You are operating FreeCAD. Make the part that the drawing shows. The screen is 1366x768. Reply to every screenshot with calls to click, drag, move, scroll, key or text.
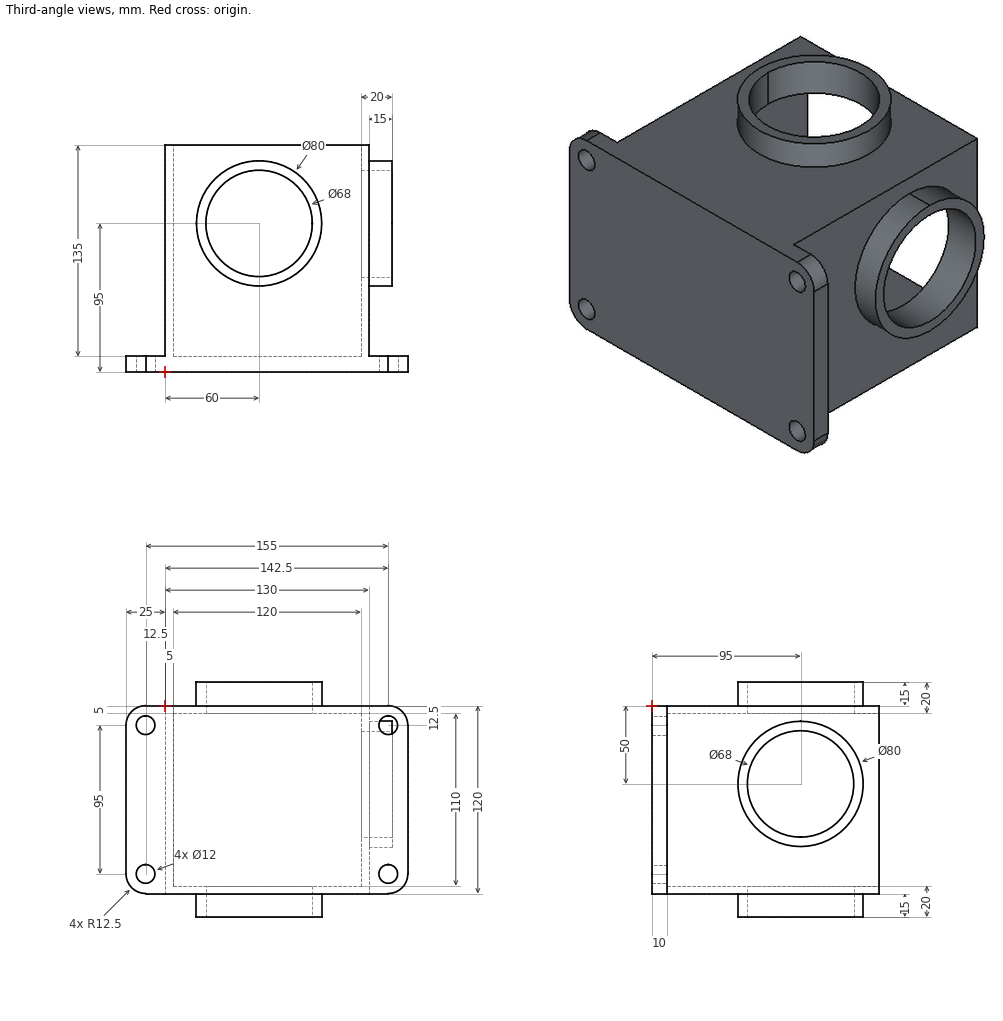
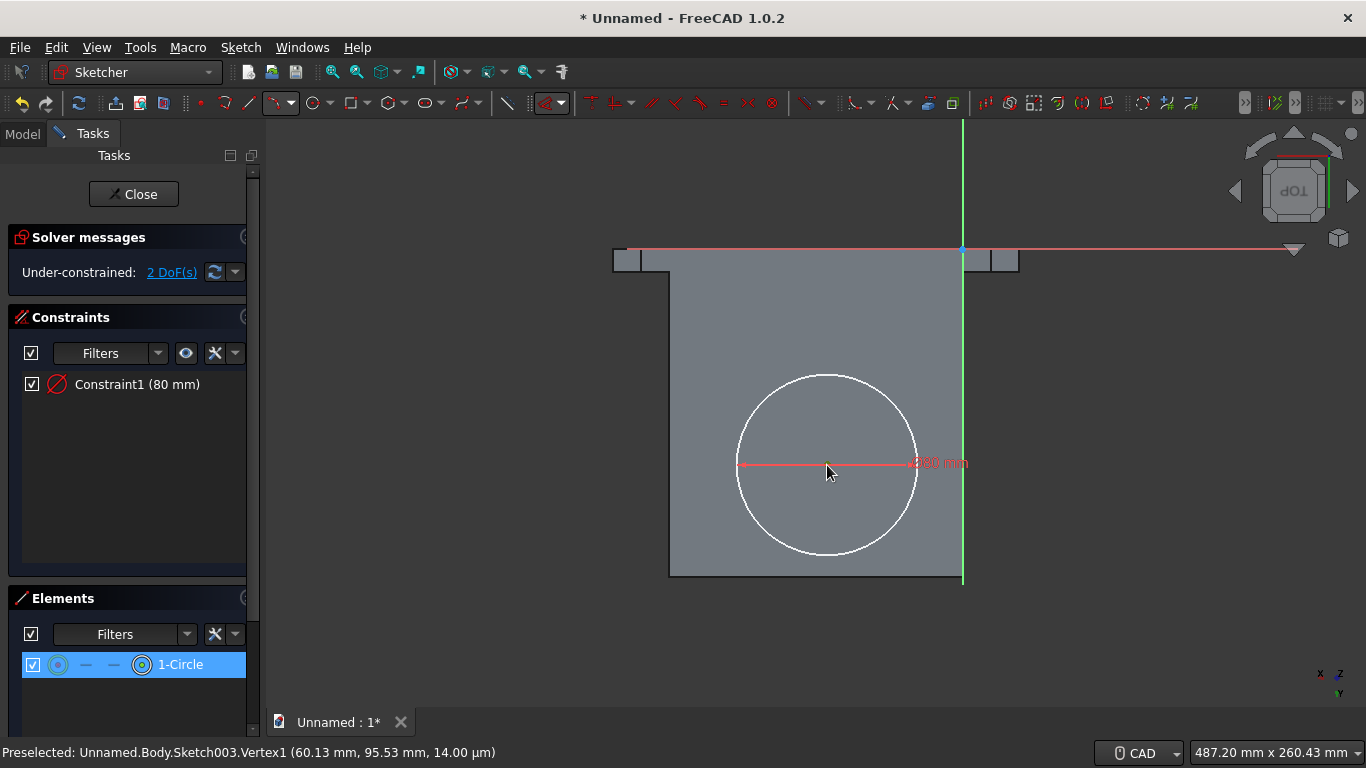
click(564, 104)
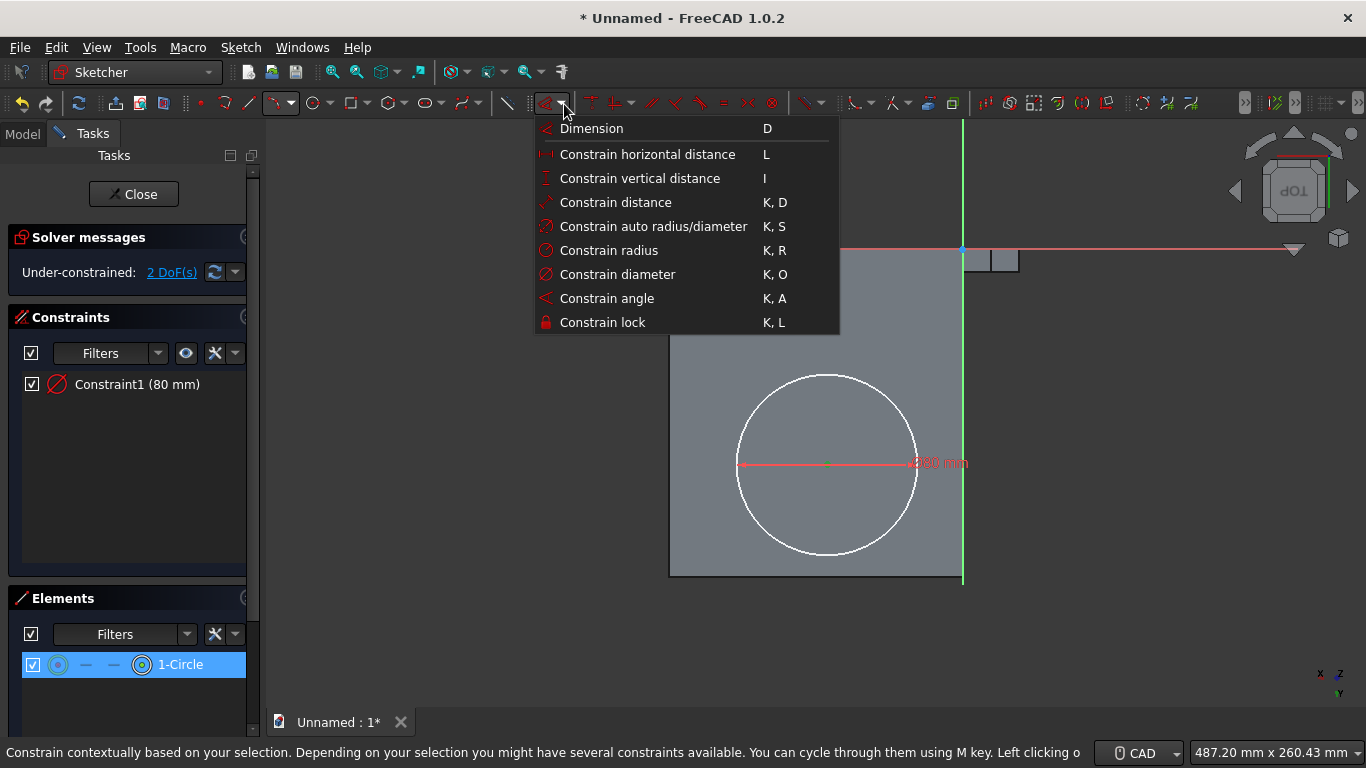
click(687, 154)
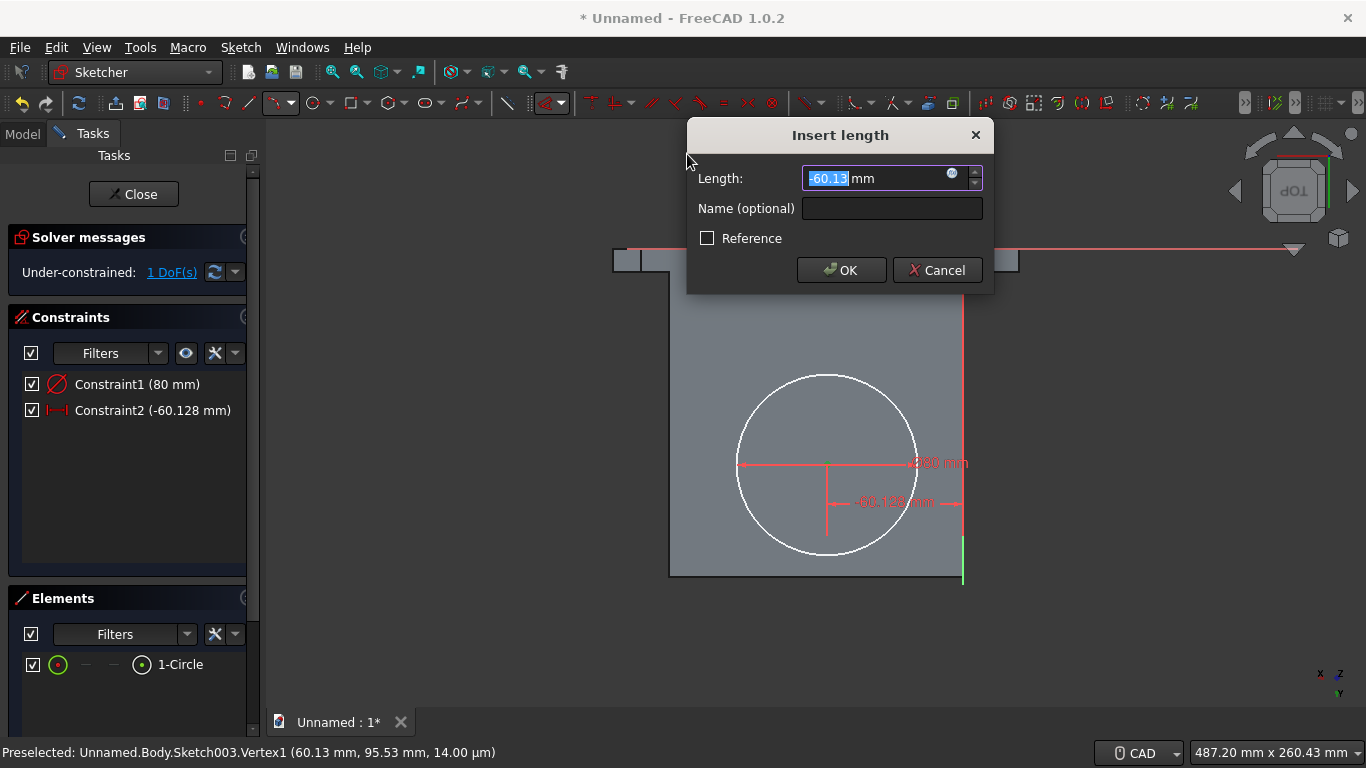
text(-60)
key(Return)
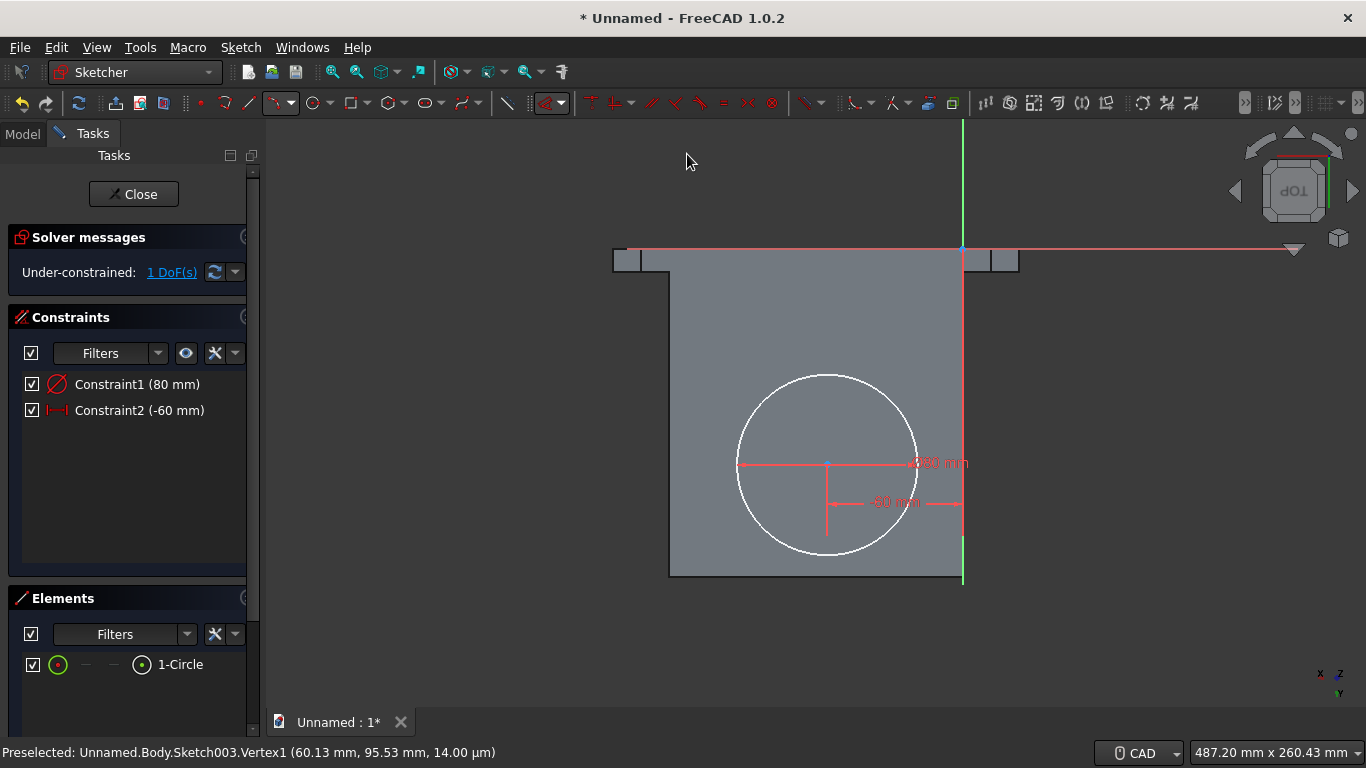
click(827, 465)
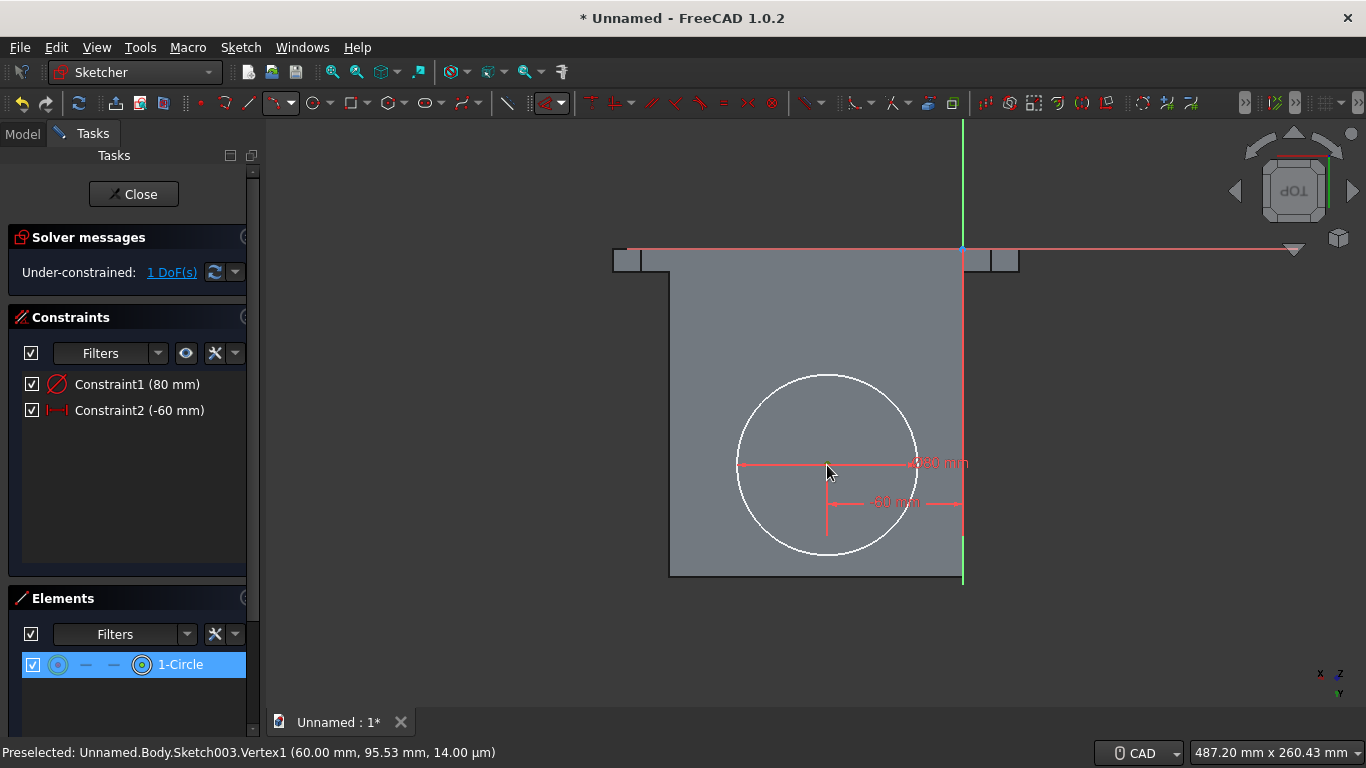
key(i)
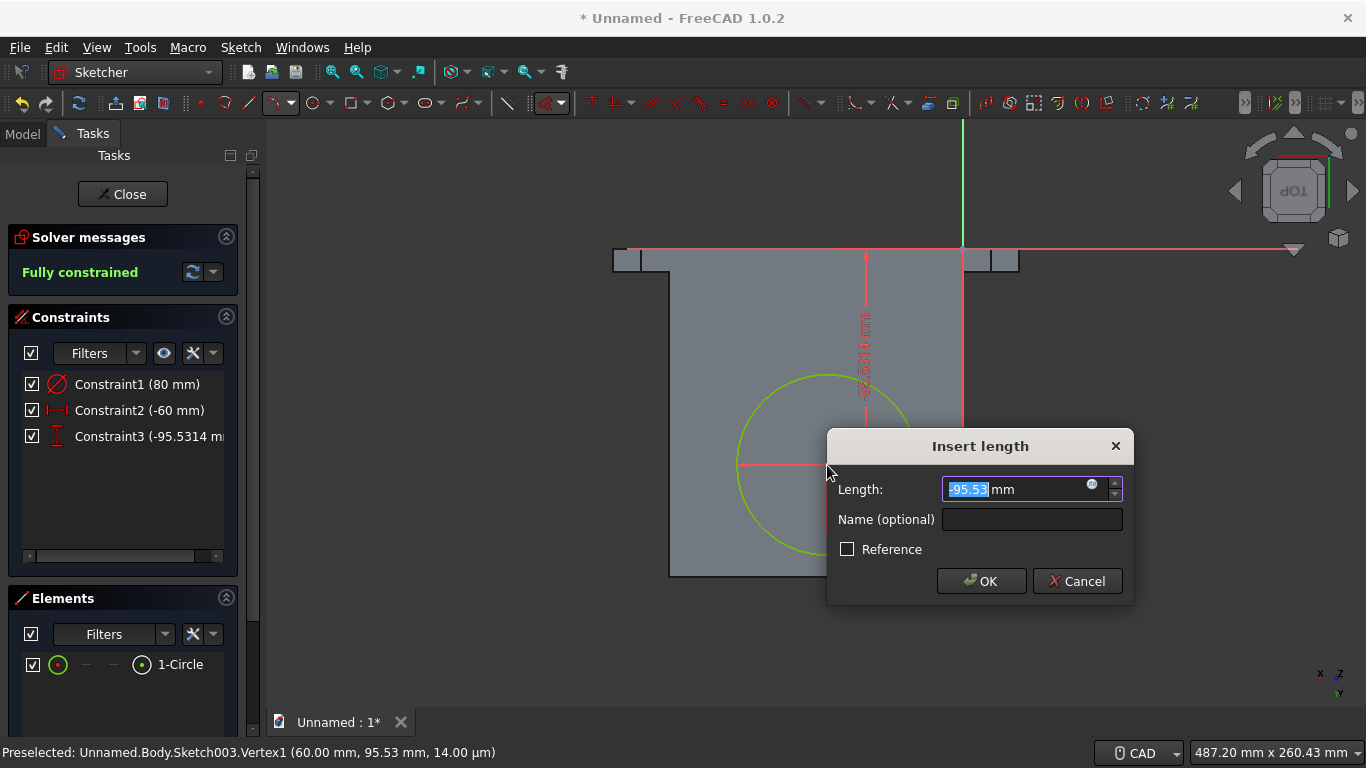
text(-95)
key(Return)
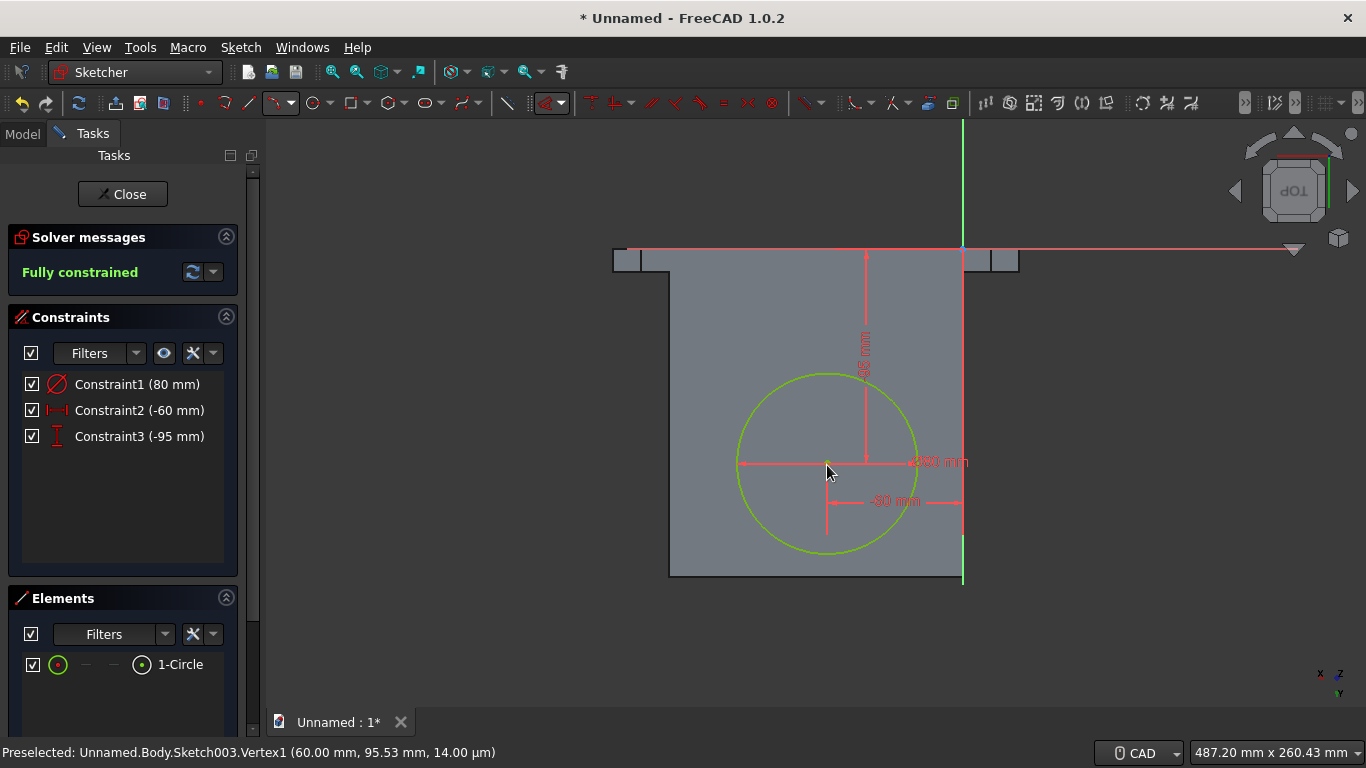
click(123, 194)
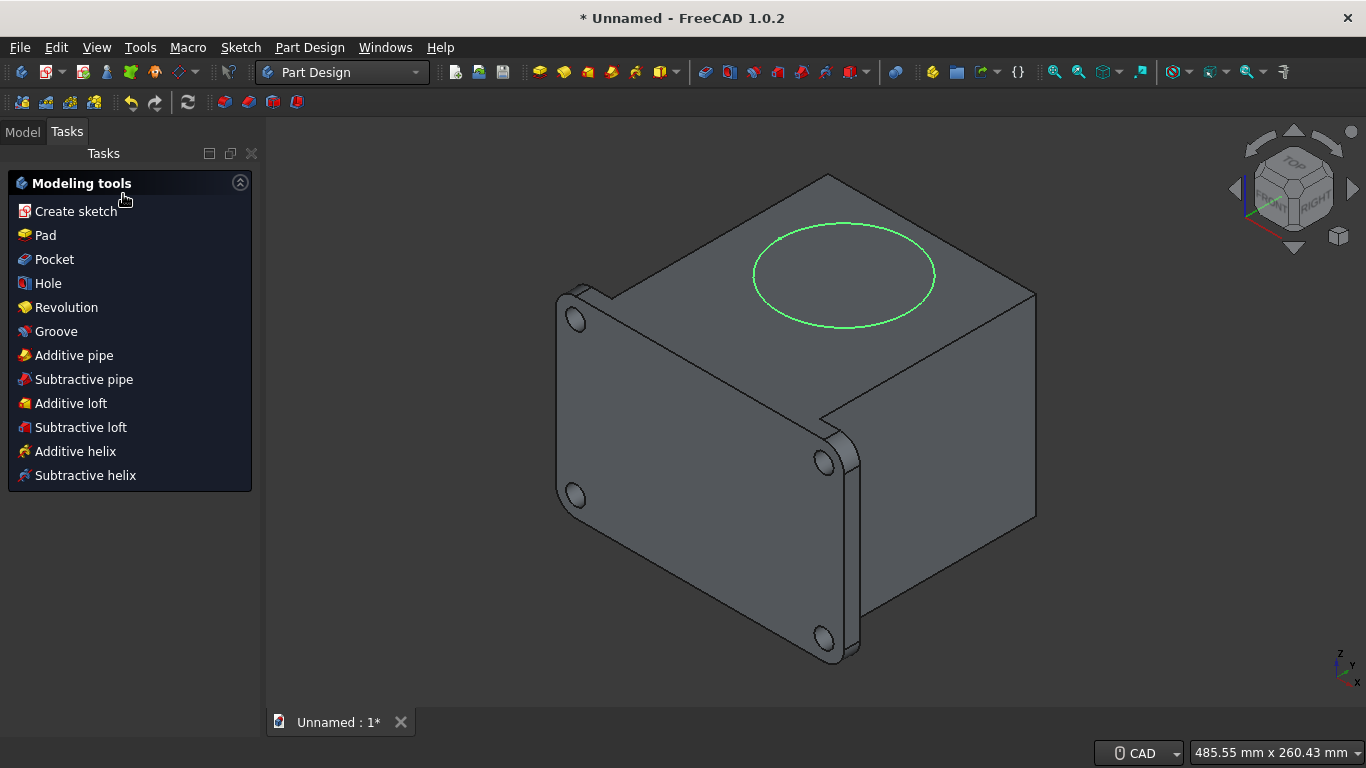
click(540, 72)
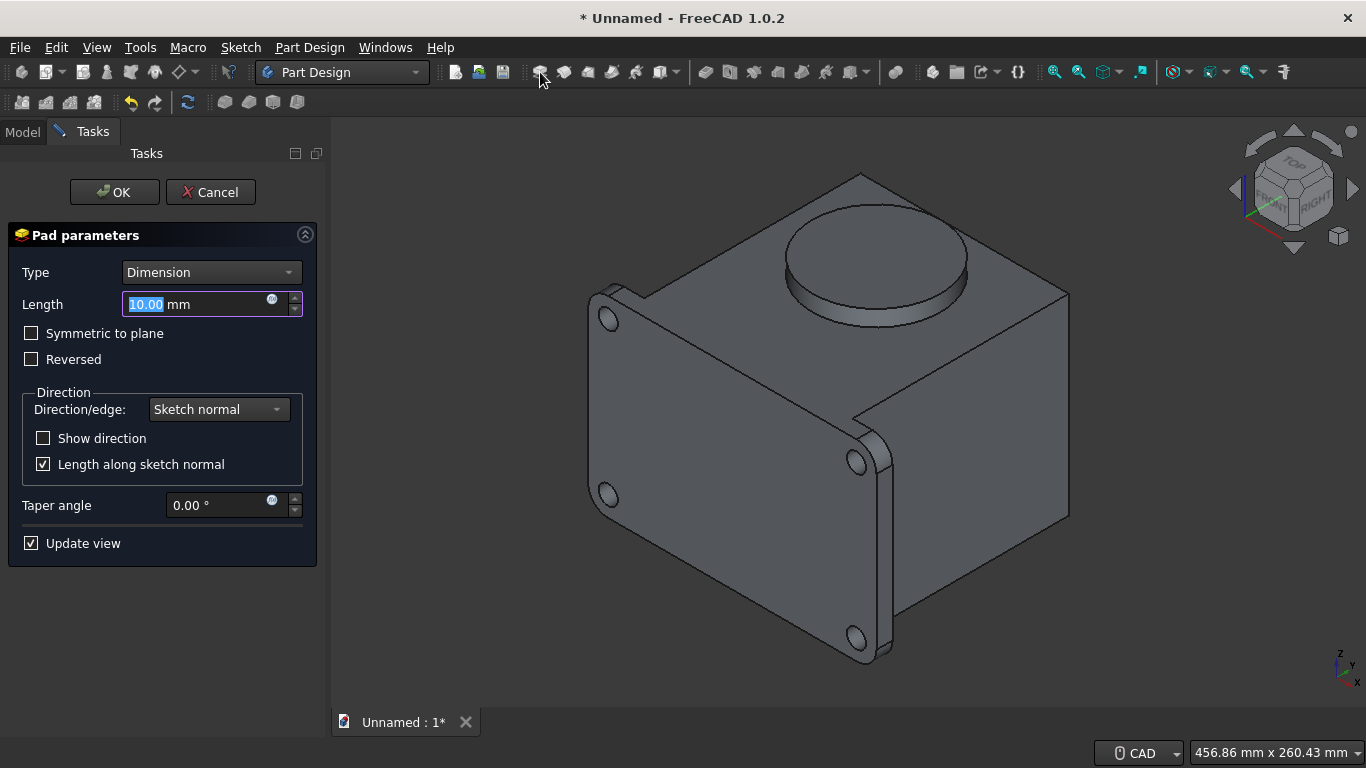
text(15)
key(Tab)